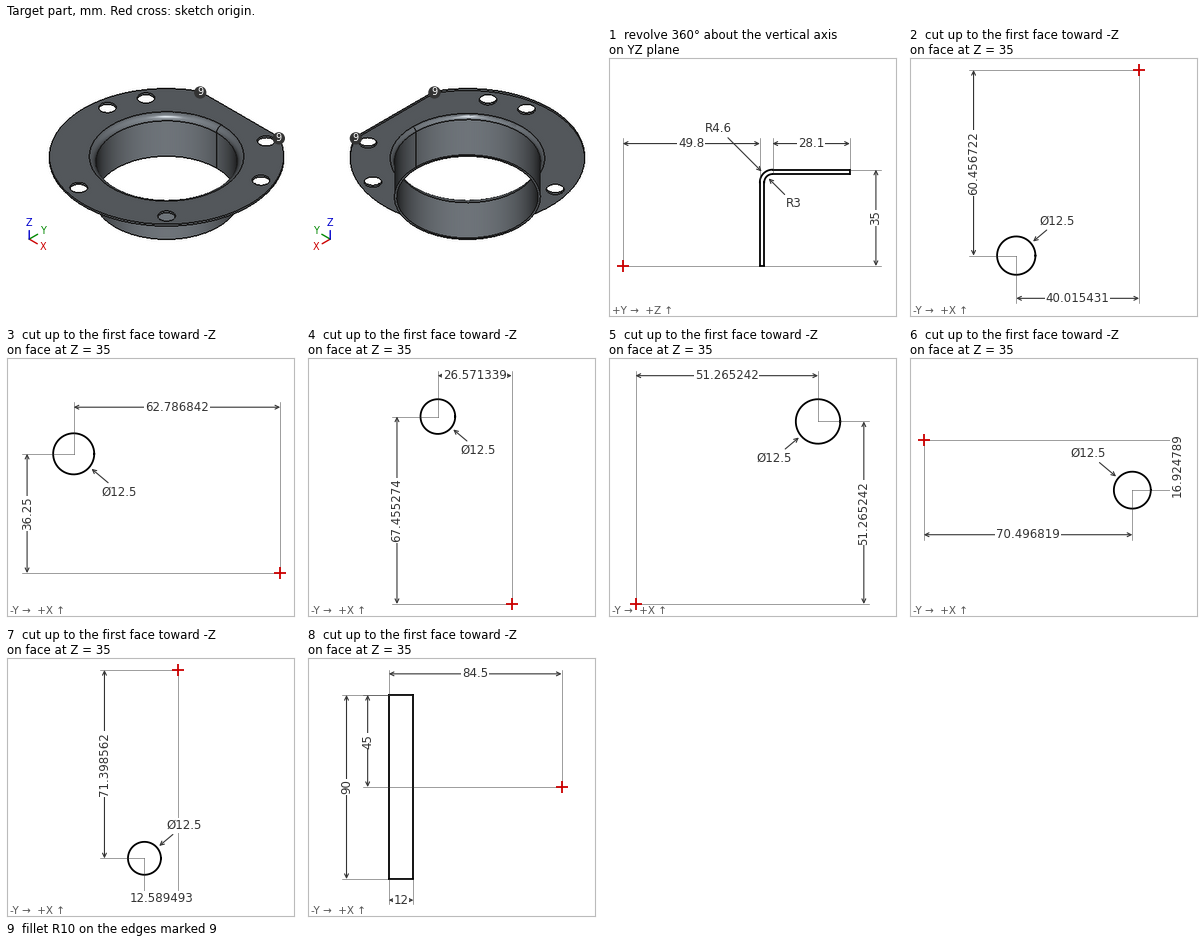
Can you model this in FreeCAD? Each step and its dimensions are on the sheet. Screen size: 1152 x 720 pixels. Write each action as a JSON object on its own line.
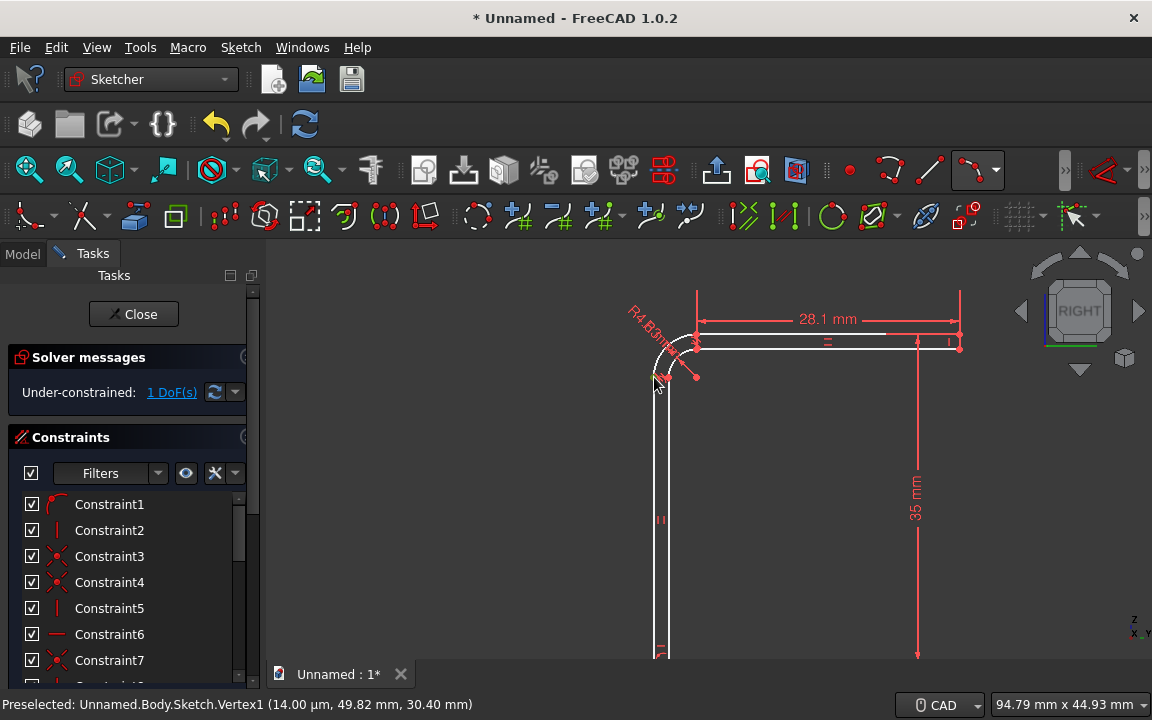
{"action": "key", "text": "l"}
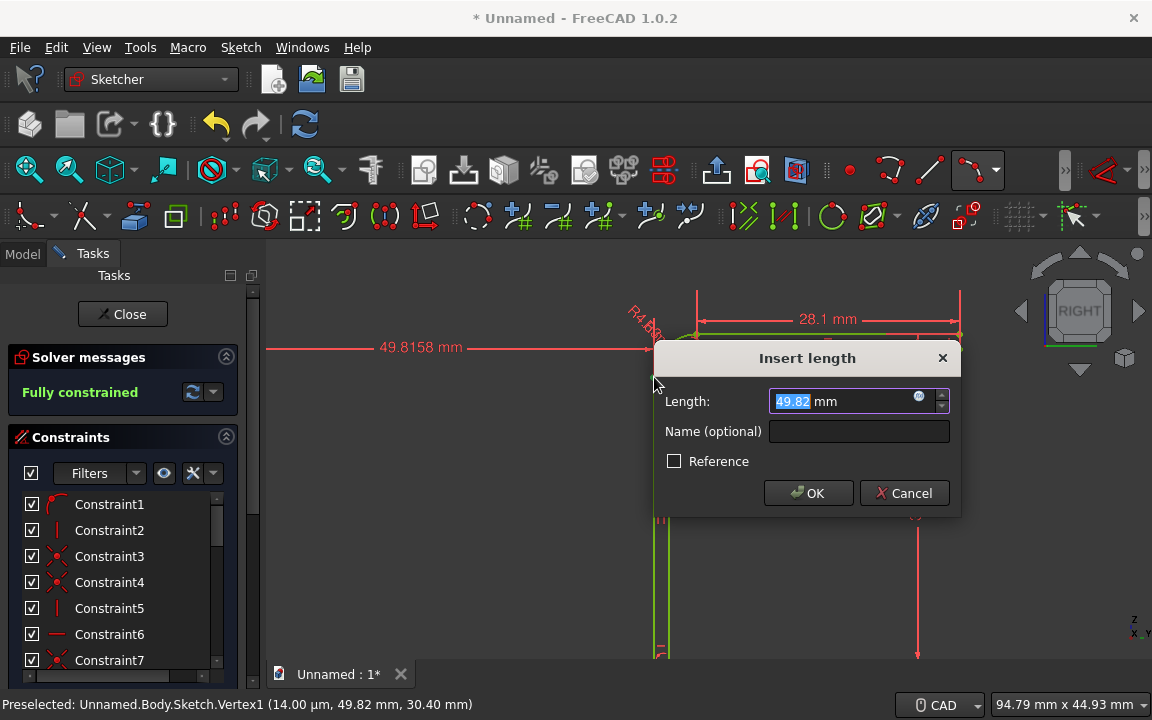
{"action": "type", "text": "49.8"}
{"action": "key", "text": "Return"}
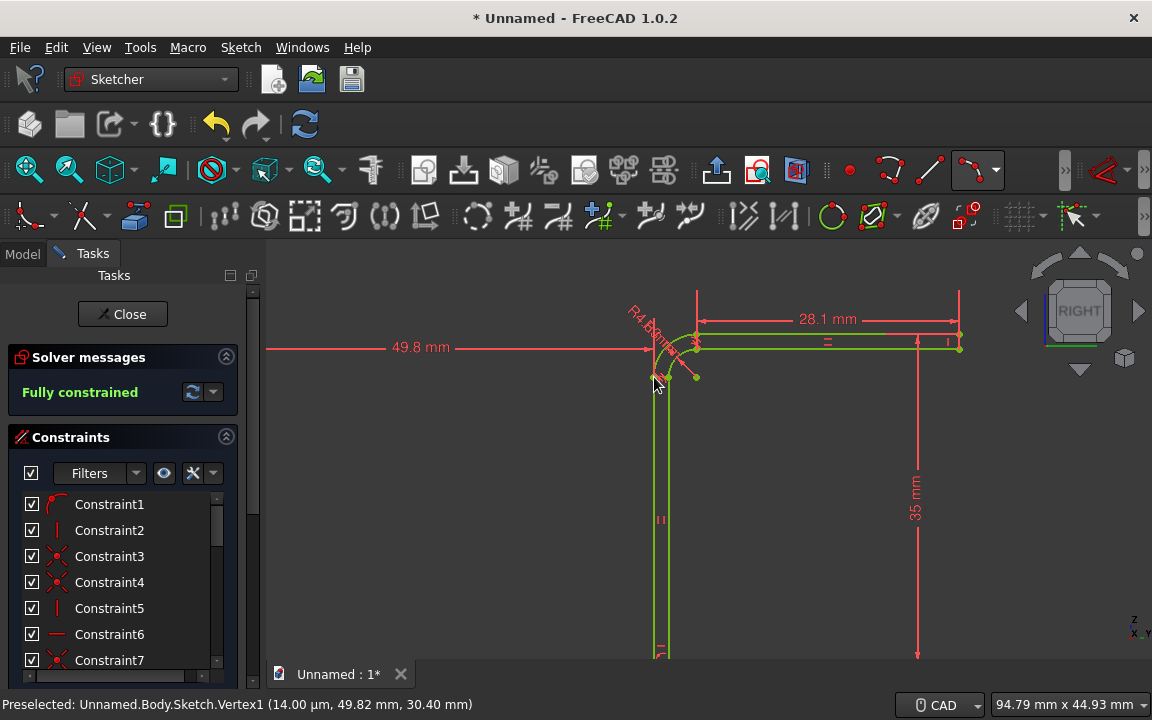
{"action": "left_click", "coordinate": [123, 314]}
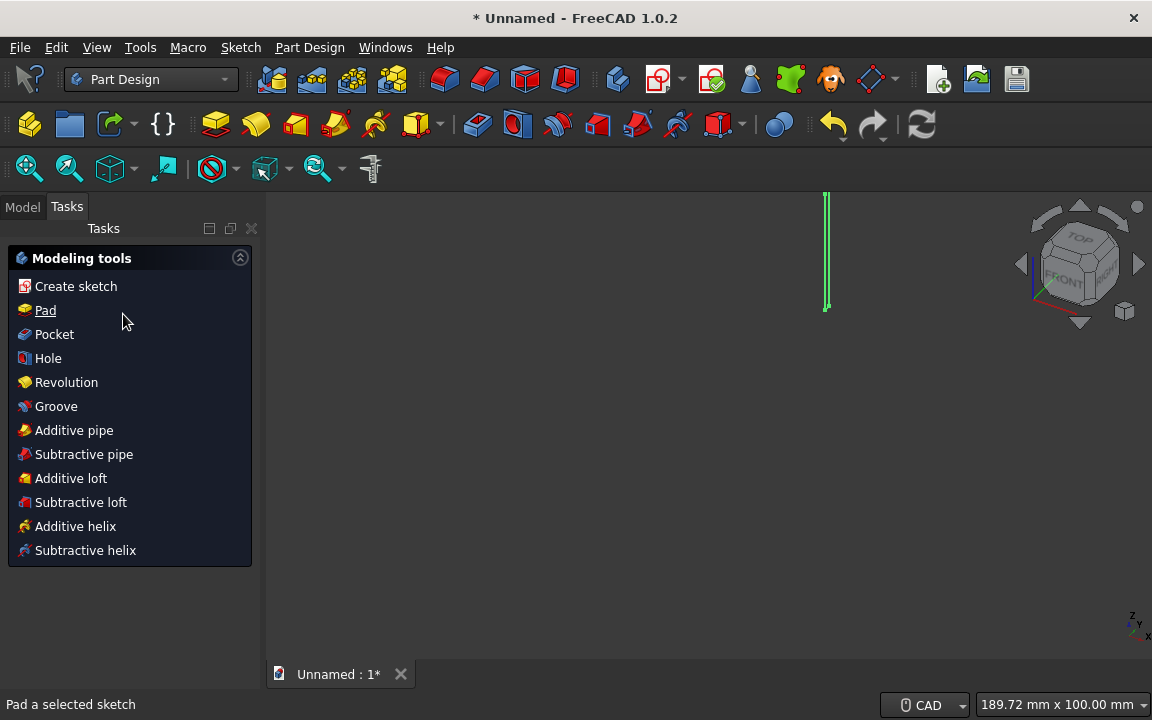
{"action": "left_click", "coordinate": [256, 124]}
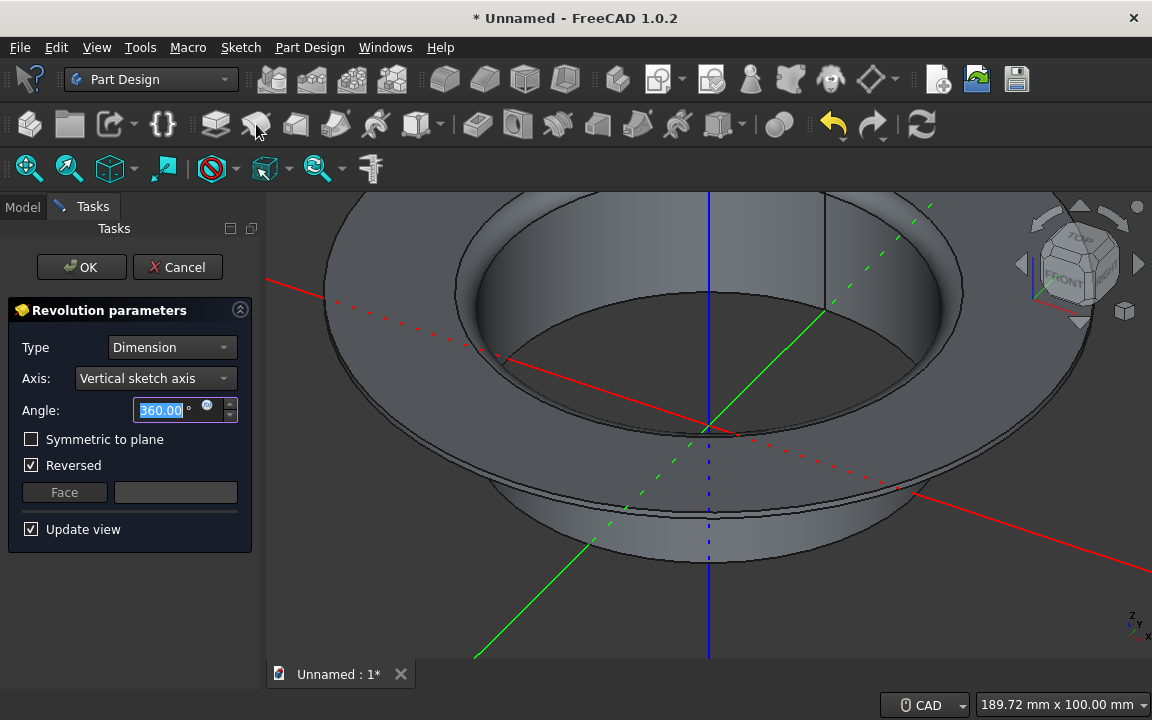
{"action": "left_click", "coordinate": [82, 267]}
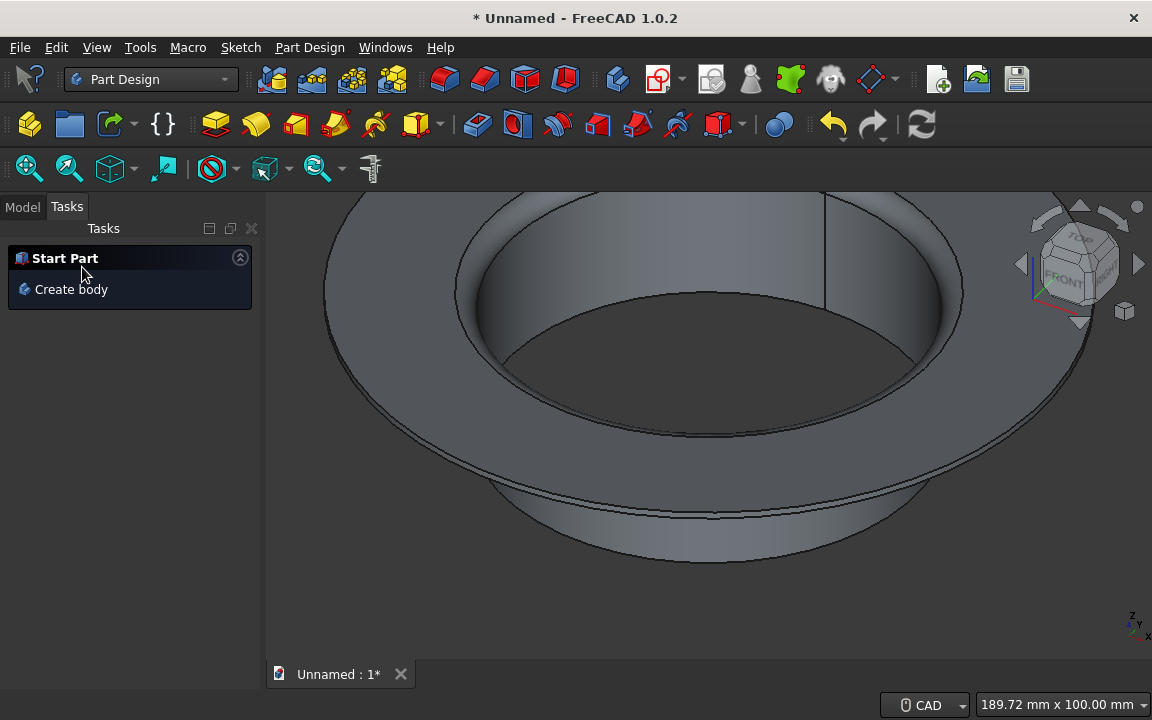
{"action": "left_click", "coordinate": [30, 170]}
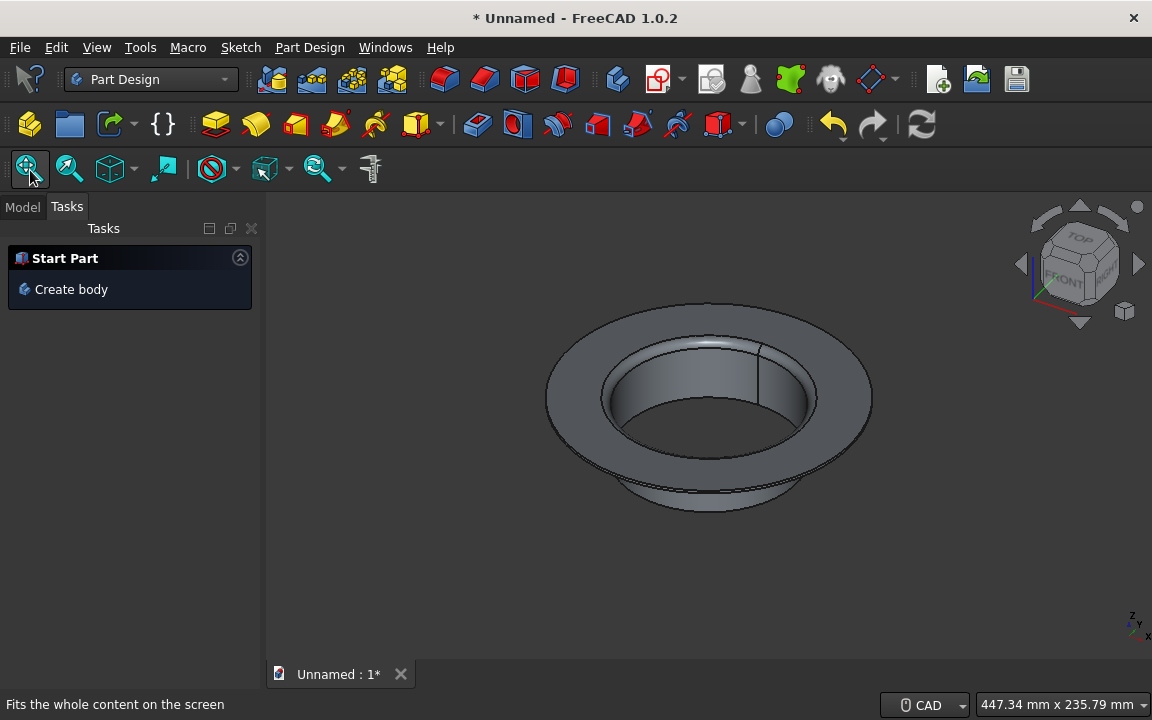
{"action": "left_click", "coordinate": [837, 377]}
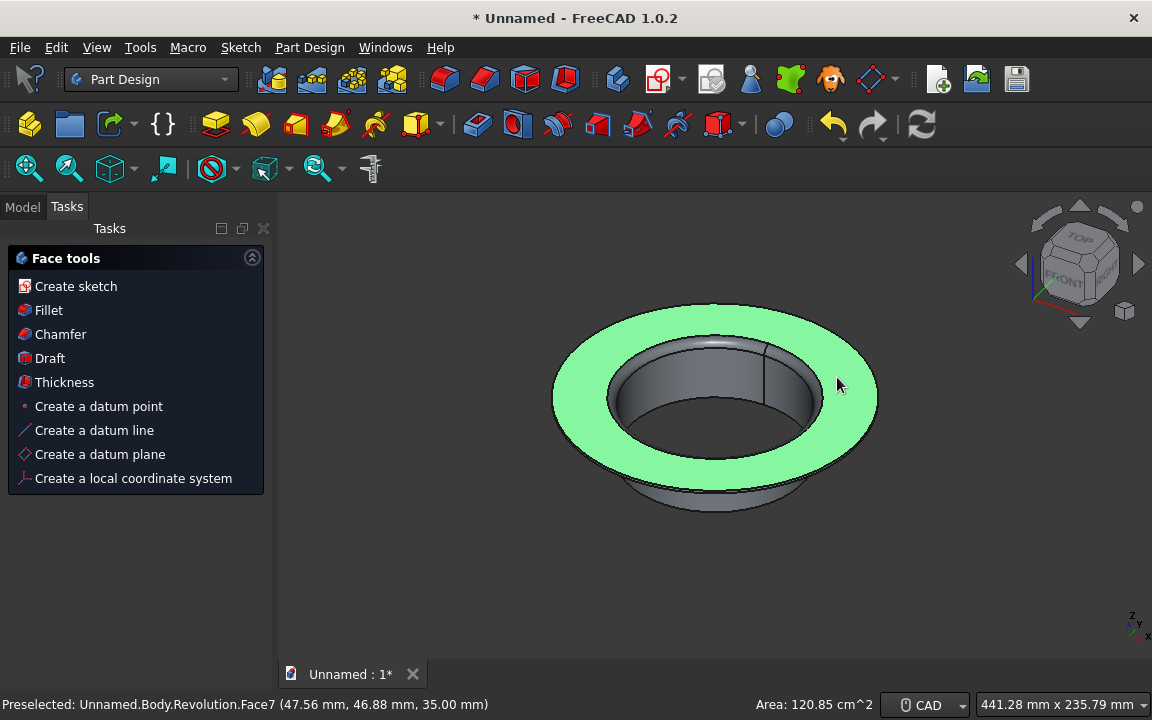
{"action": "left_click", "coordinate": [658, 80]}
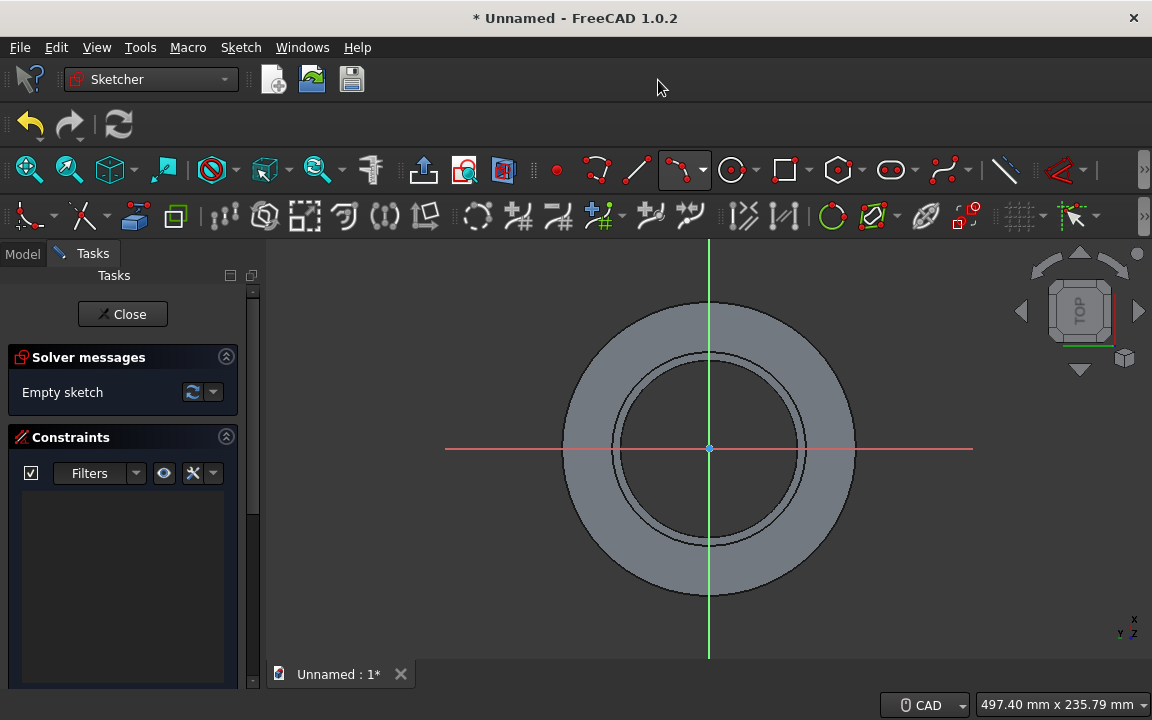
{"action": "scroll", "coordinate": [637, 567], "scroll_direction": "up", "scroll_amount": 12}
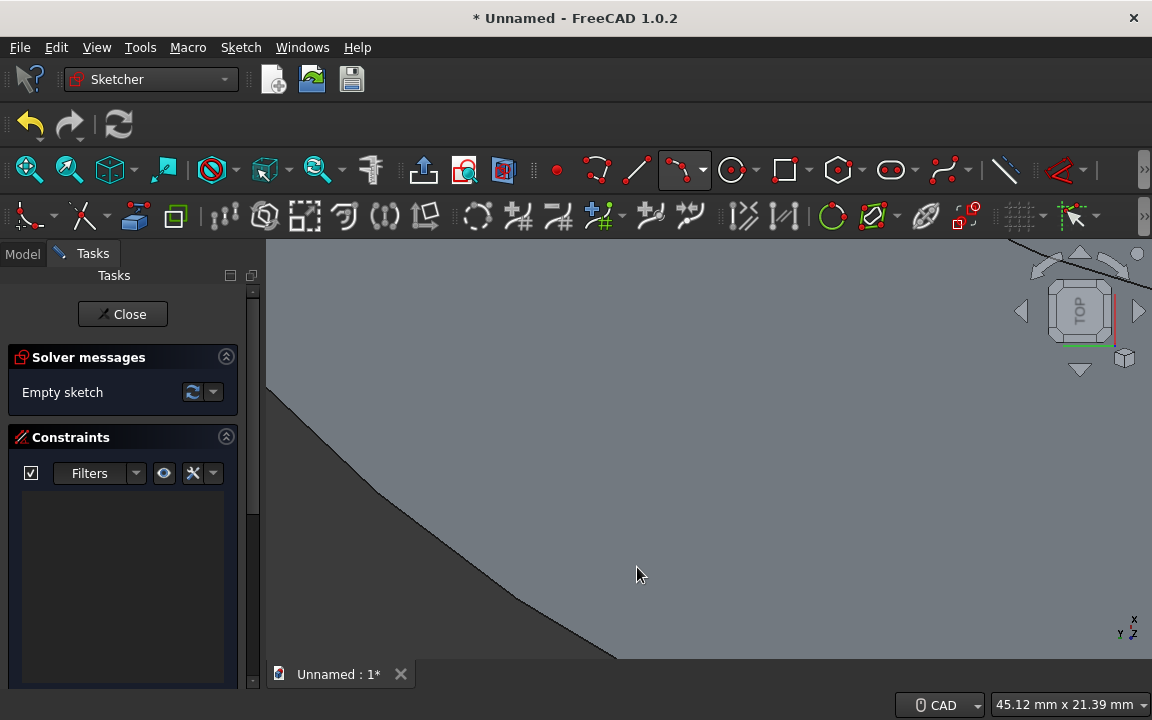
{"action": "key", "text": "g c"}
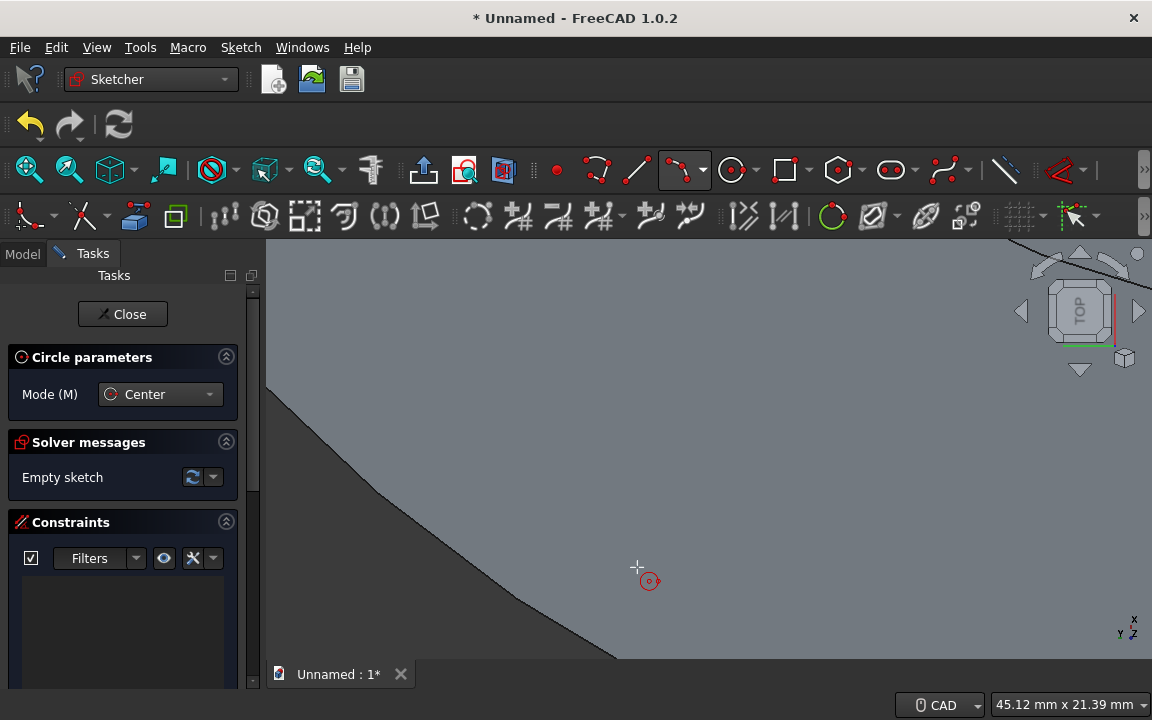
{"action": "left_click", "coordinate": [641, 446]}
{"action": "mouse_move", "coordinate": [728, 359]}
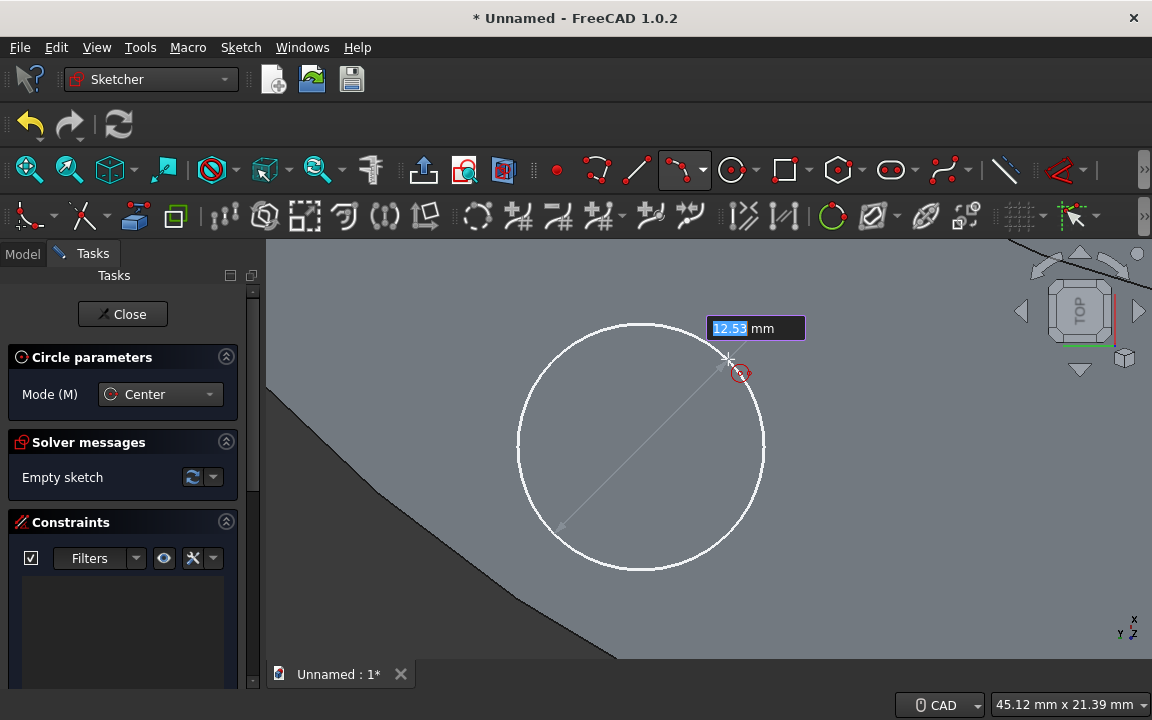
{"action": "type", "text": "12.5"}
{"action": "key", "text": "Return"}
{"action": "key", "text": "Escape"}